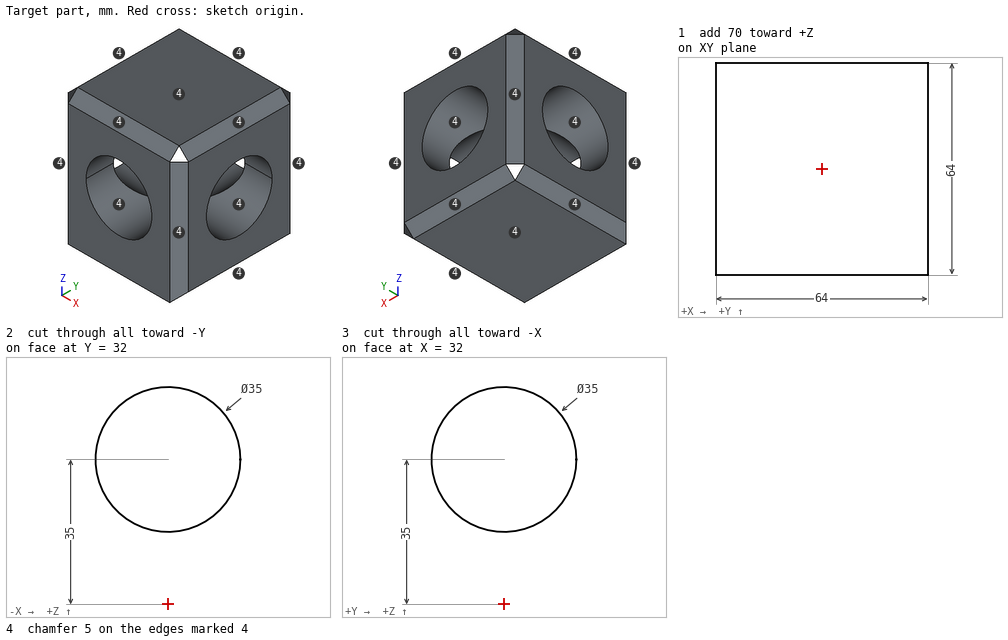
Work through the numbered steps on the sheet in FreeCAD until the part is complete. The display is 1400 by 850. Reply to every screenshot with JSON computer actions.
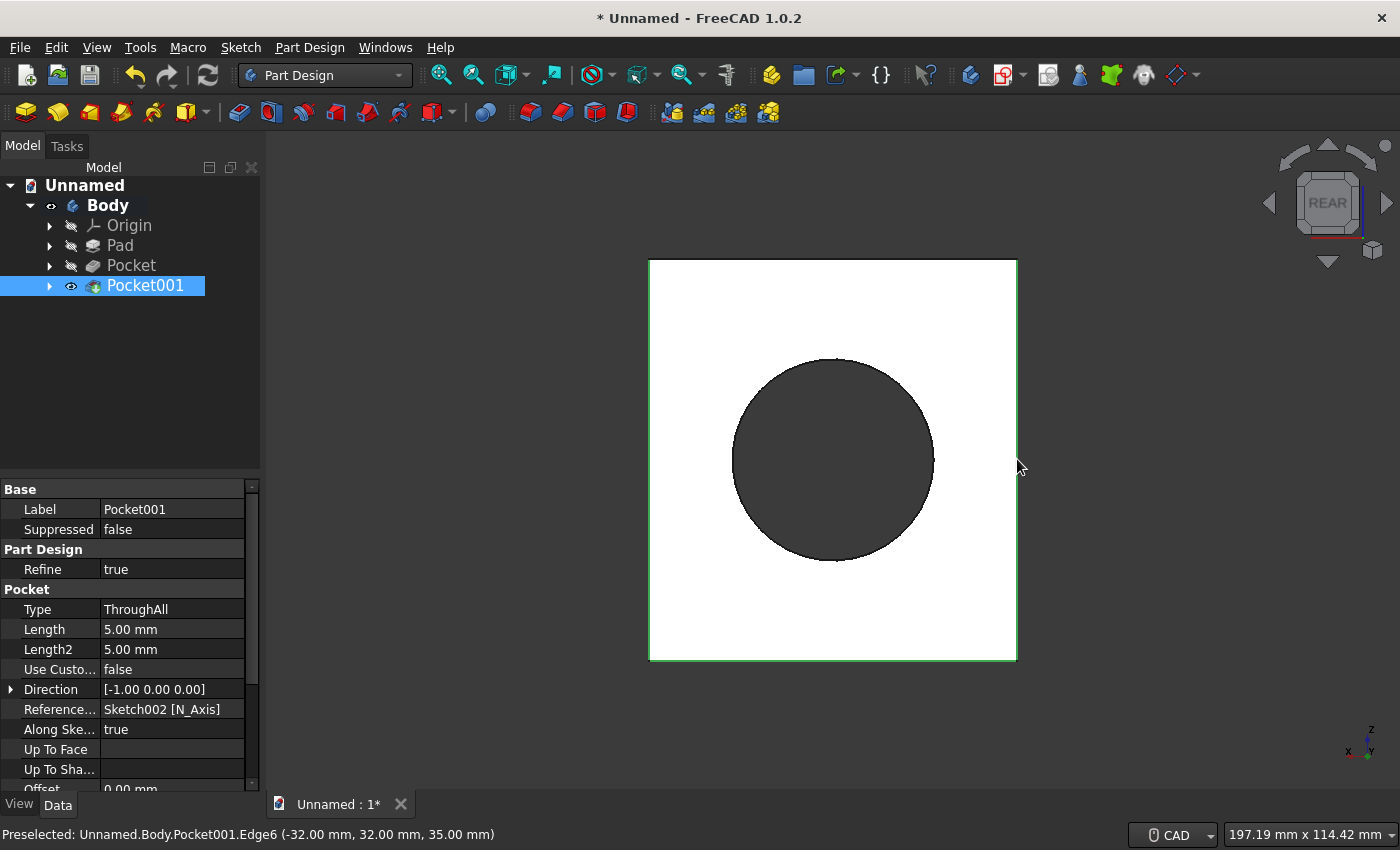
{"action": "left_click", "coordinate": [564, 112]}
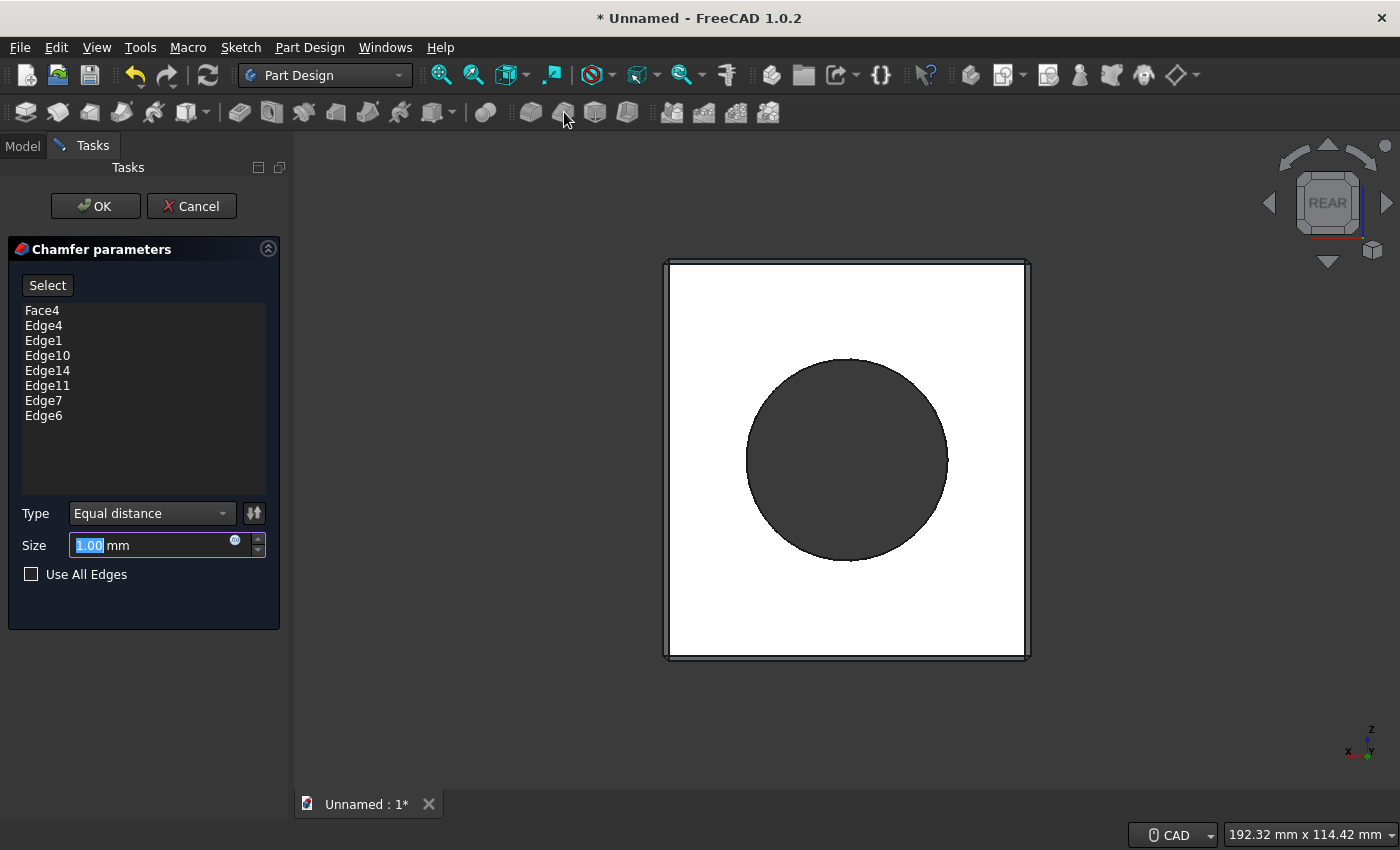
{"action": "type", "text": "5"}
{"action": "key", "text": "Tab"}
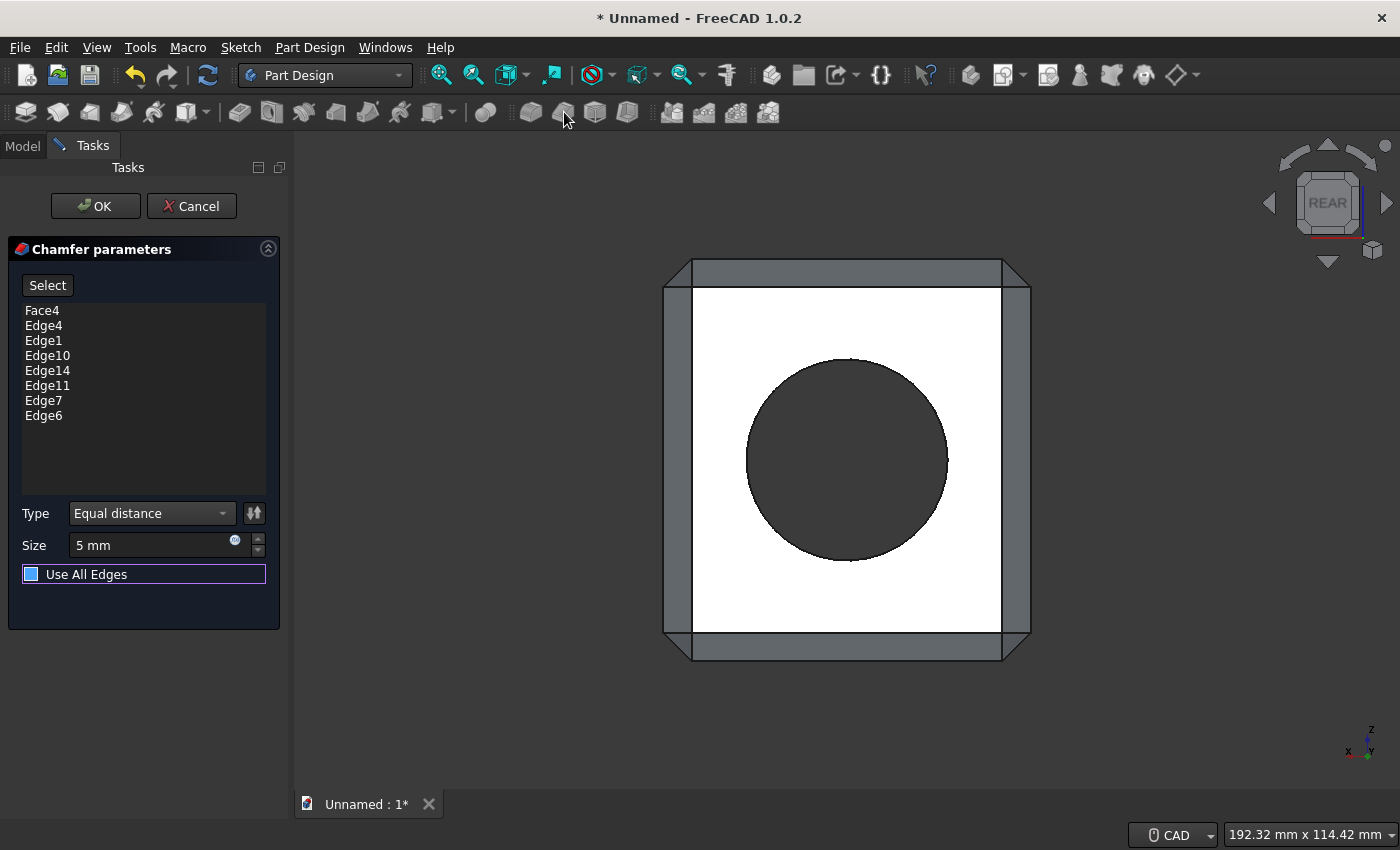
{"action": "left_click", "coordinate": [96, 206]}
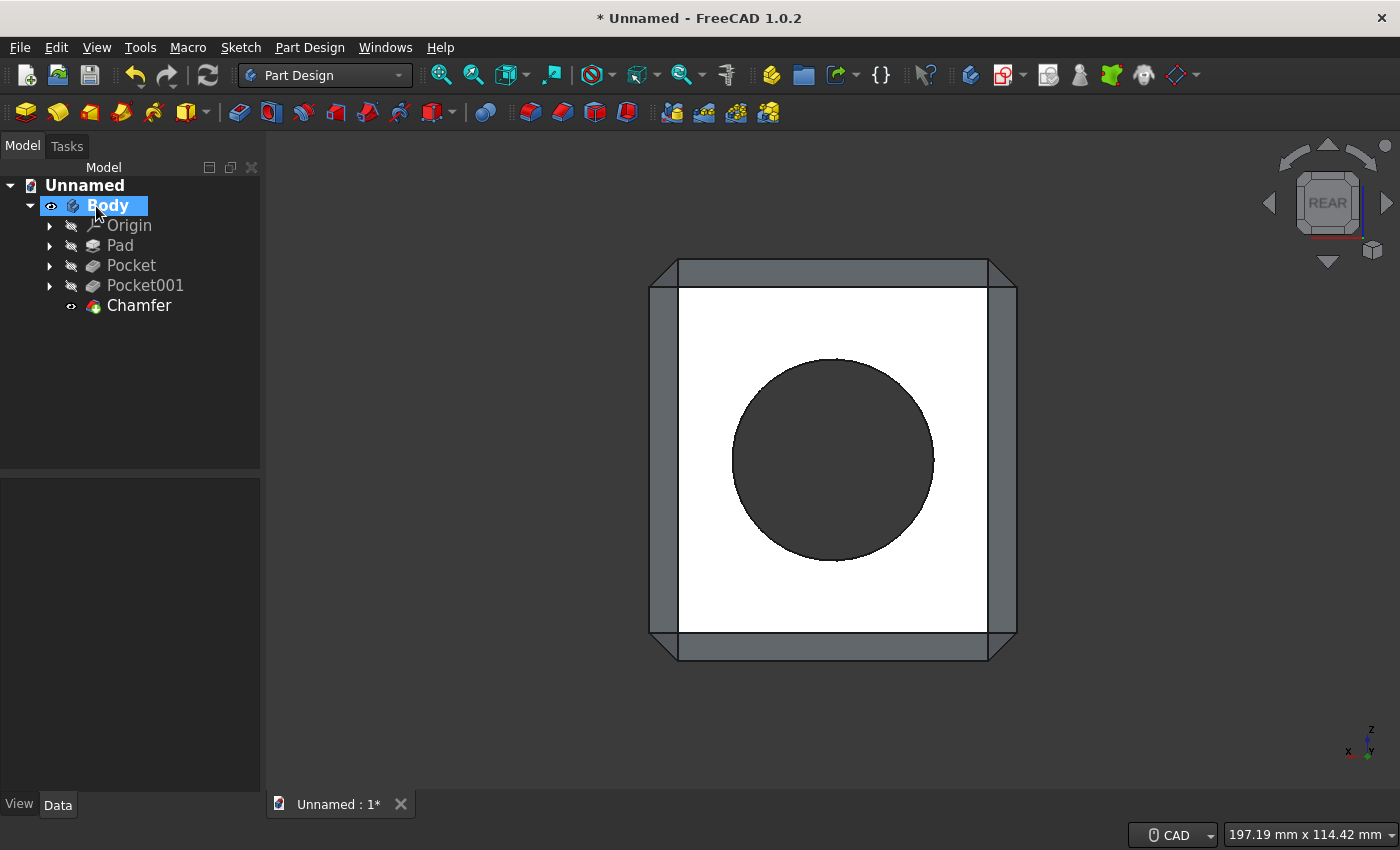
{"action": "key", "text": "0"}